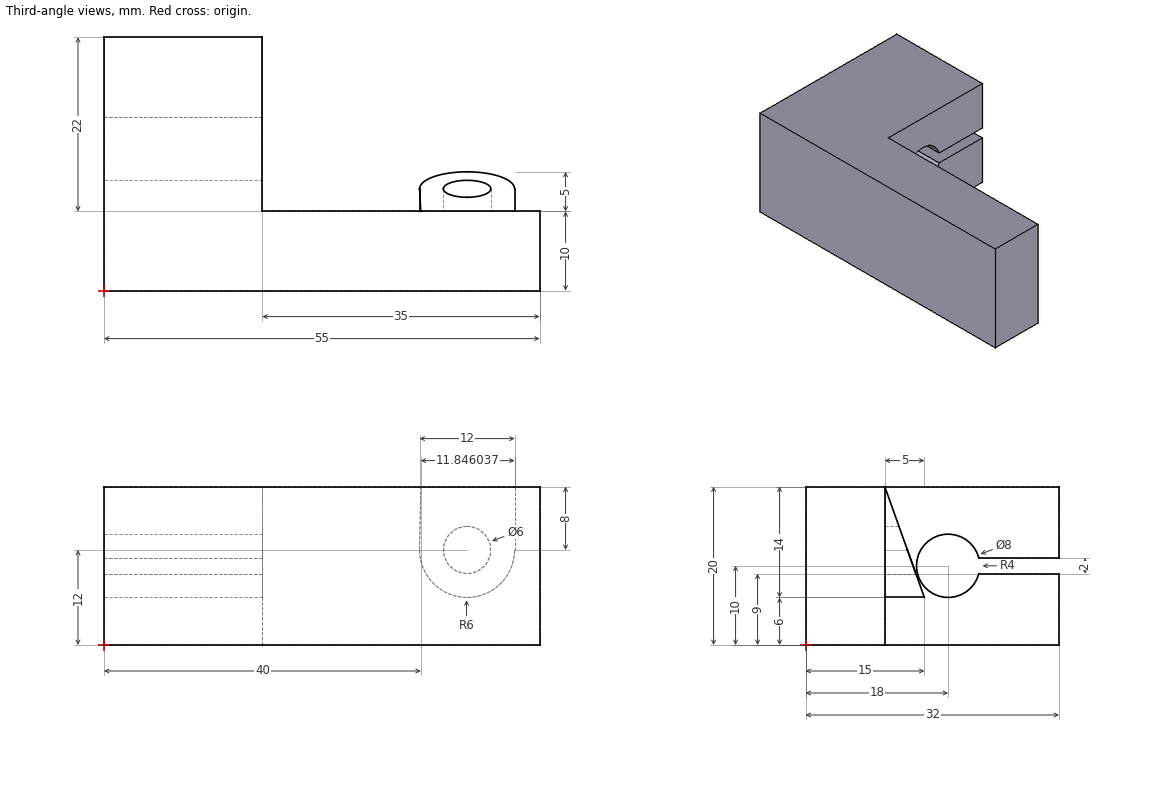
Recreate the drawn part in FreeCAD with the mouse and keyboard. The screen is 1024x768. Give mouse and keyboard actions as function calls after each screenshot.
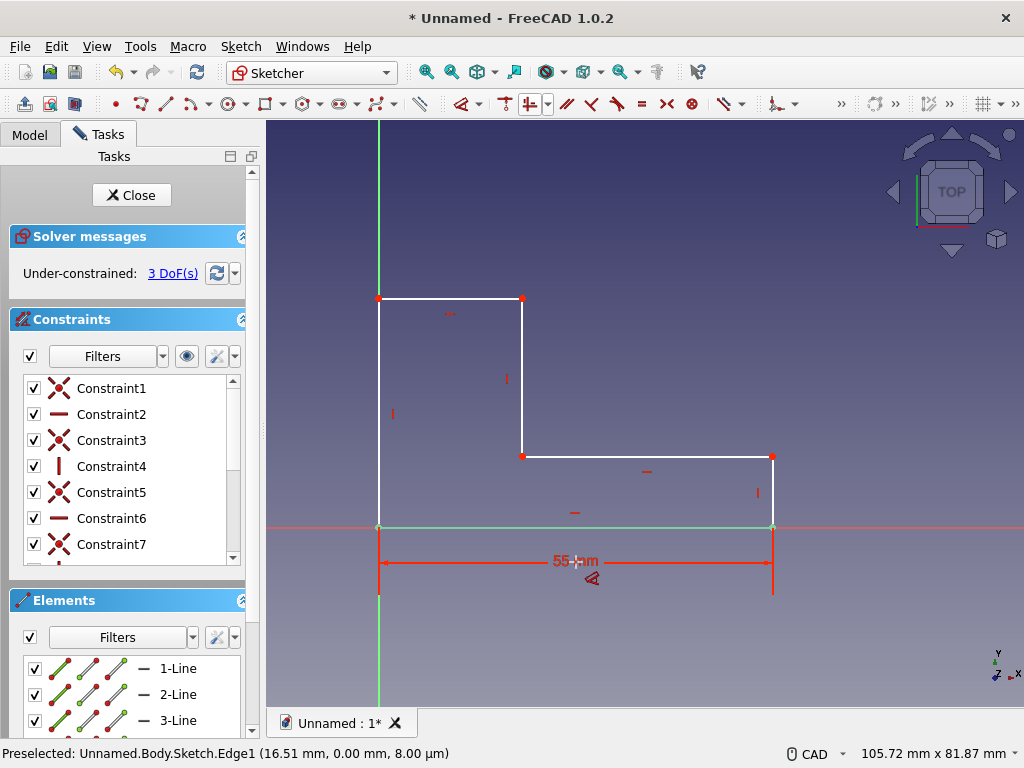
click(773, 506)
click(807, 492)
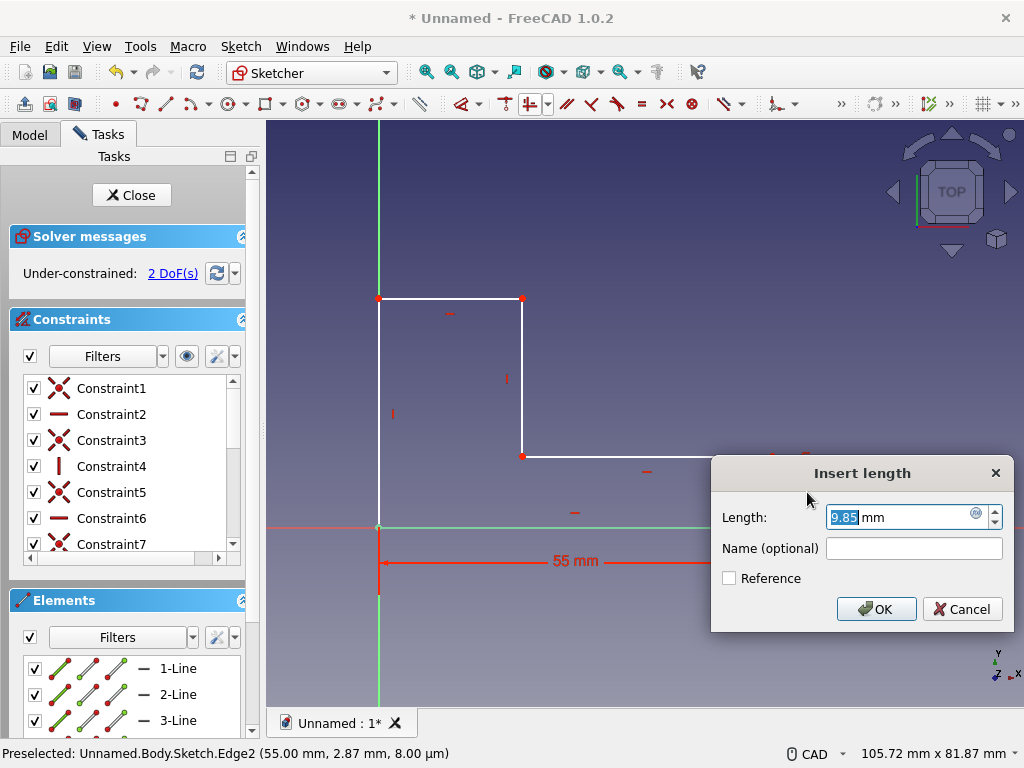
text(10)
key(Return)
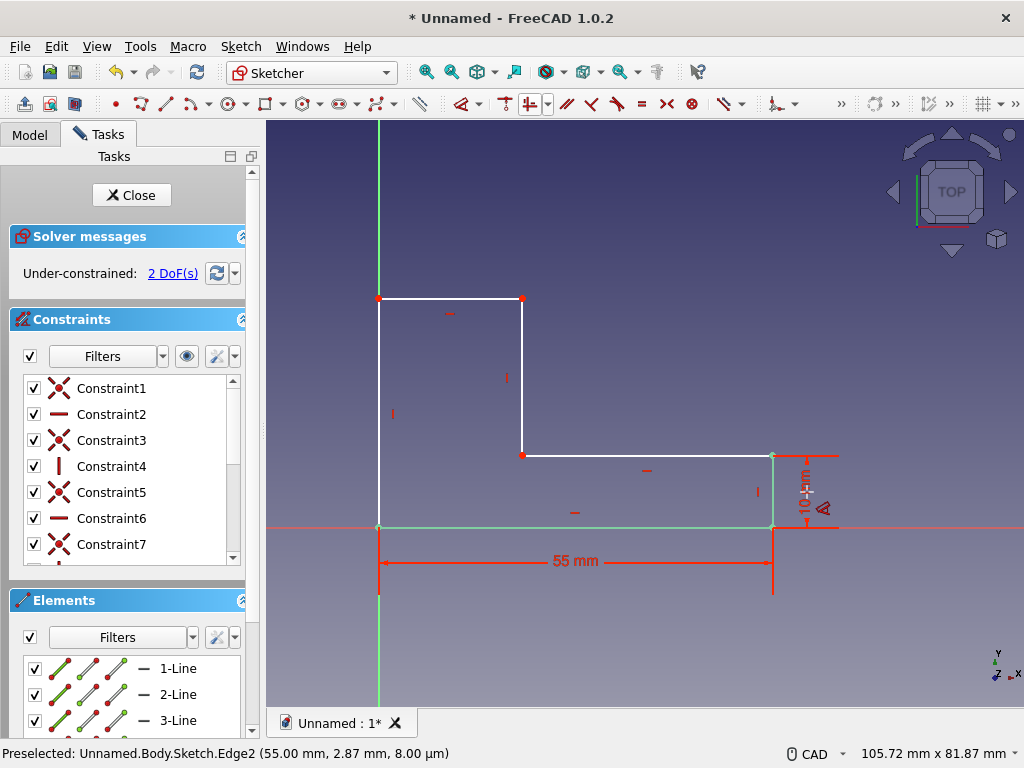
click(698, 456)
click(647, 490)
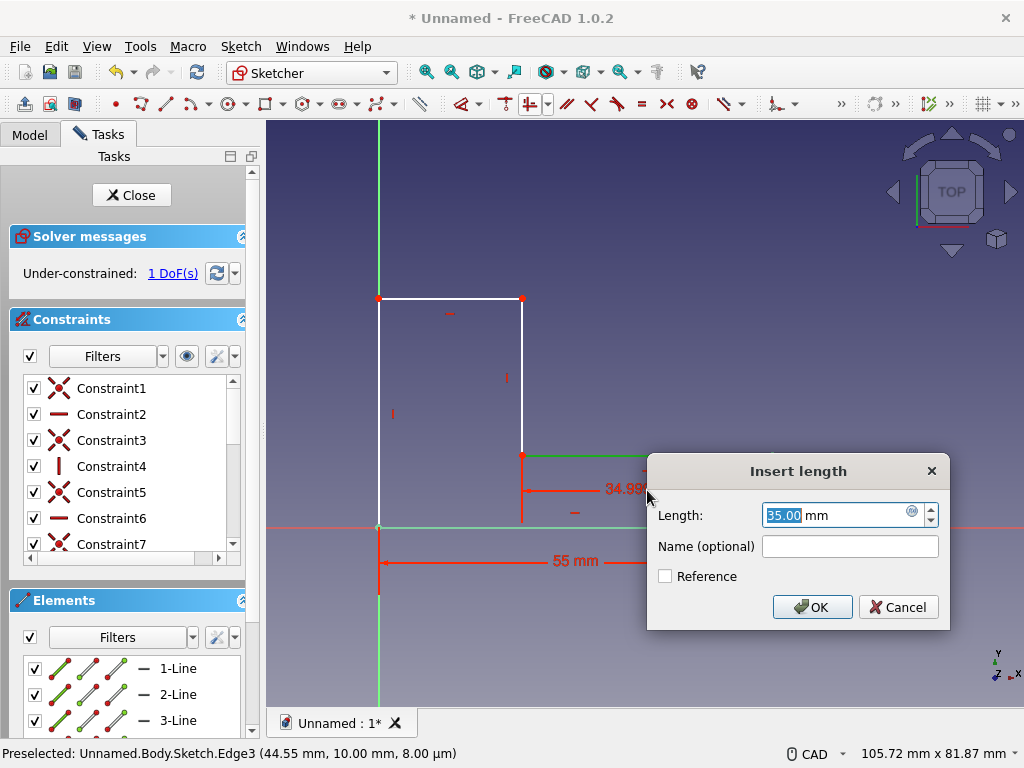
text(35)
key(Return)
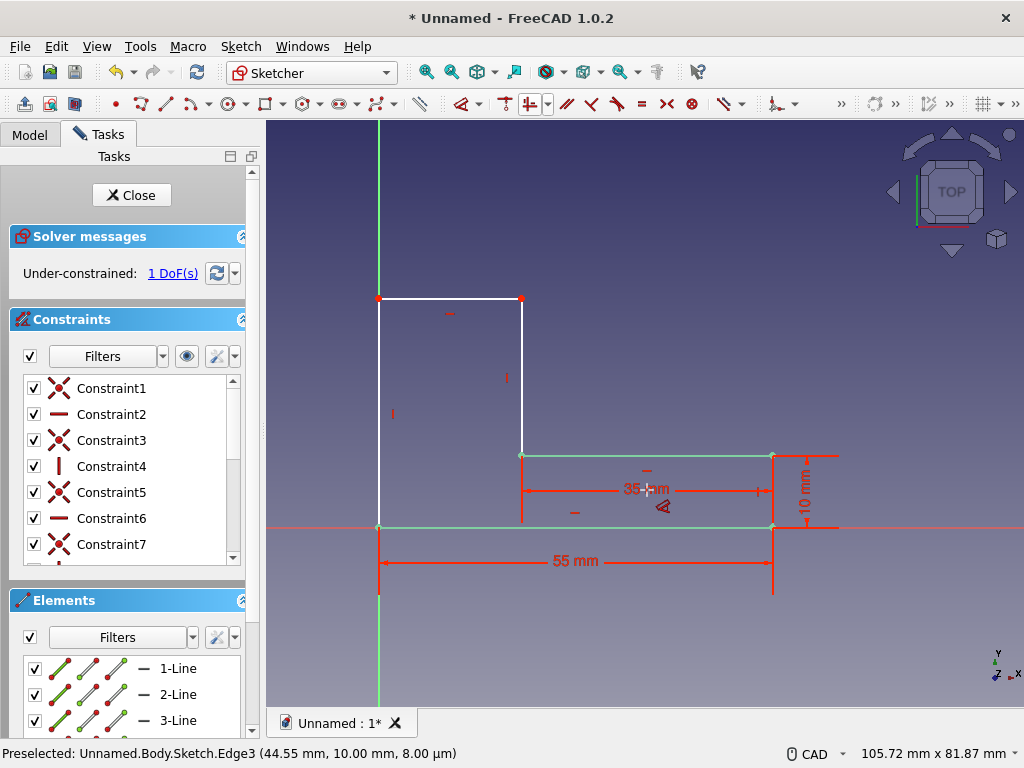
click(522, 409)
click(488, 377)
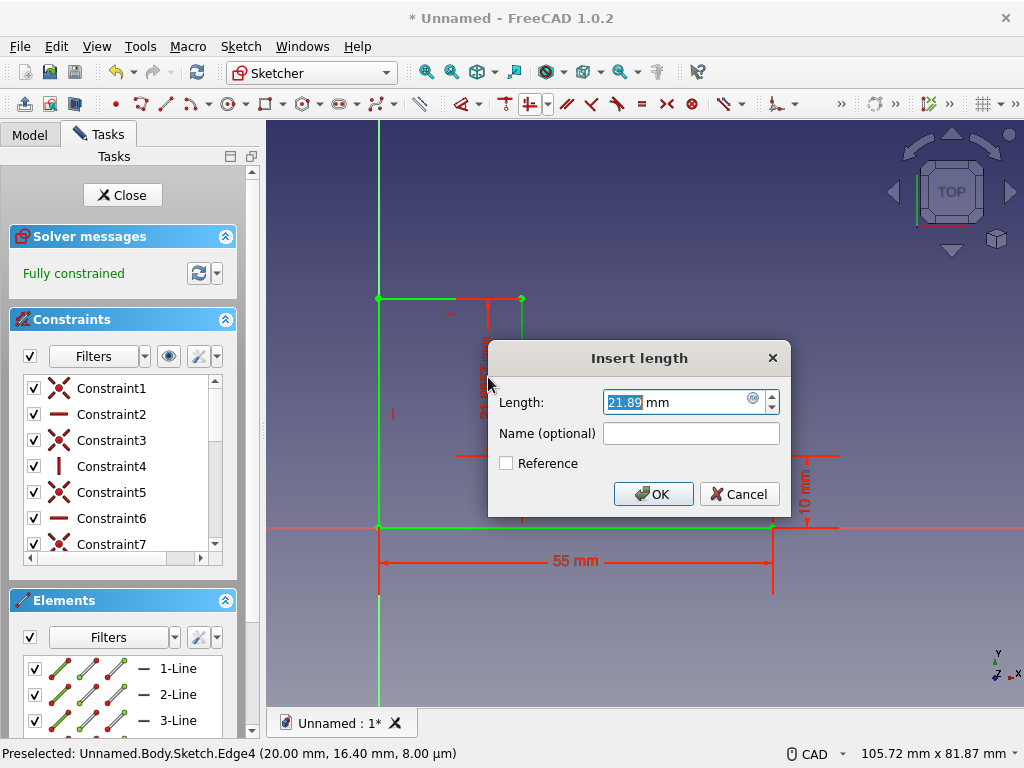
text(22)
key(Return)
key(Escape)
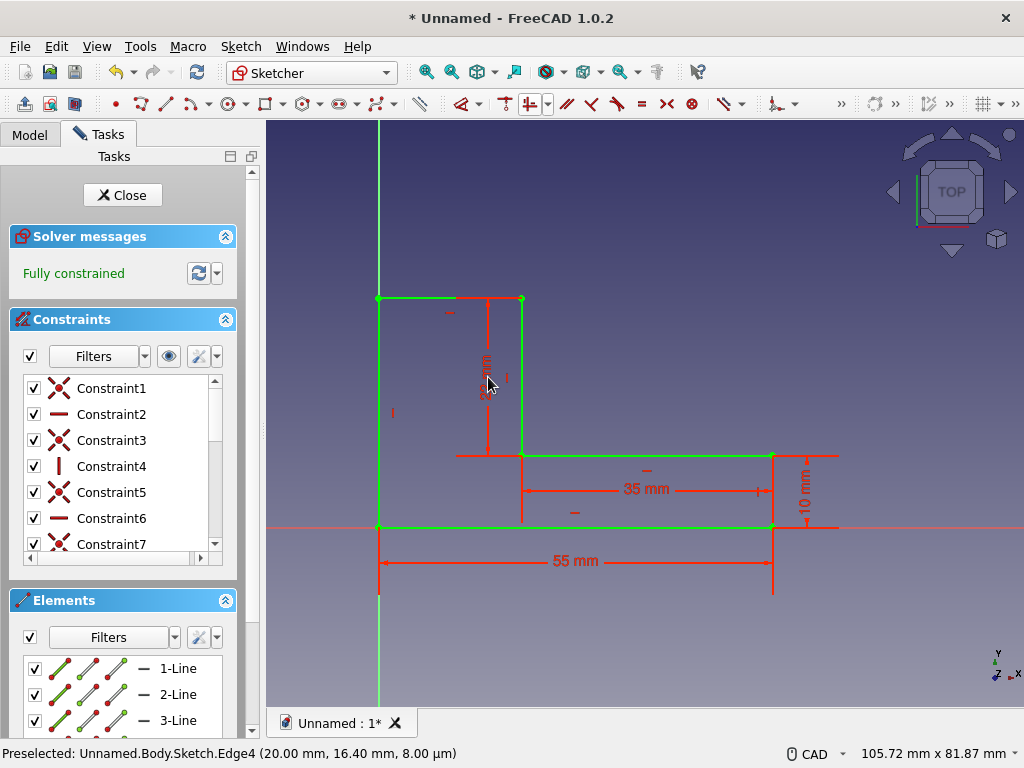
click(123, 195)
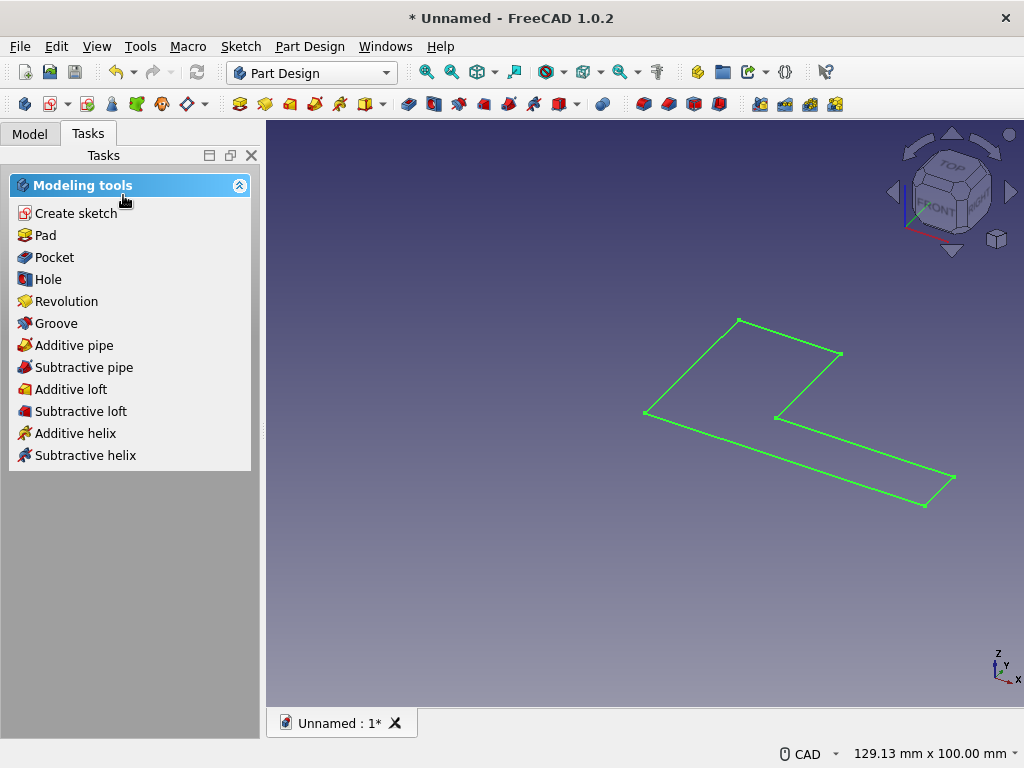
click(240, 104)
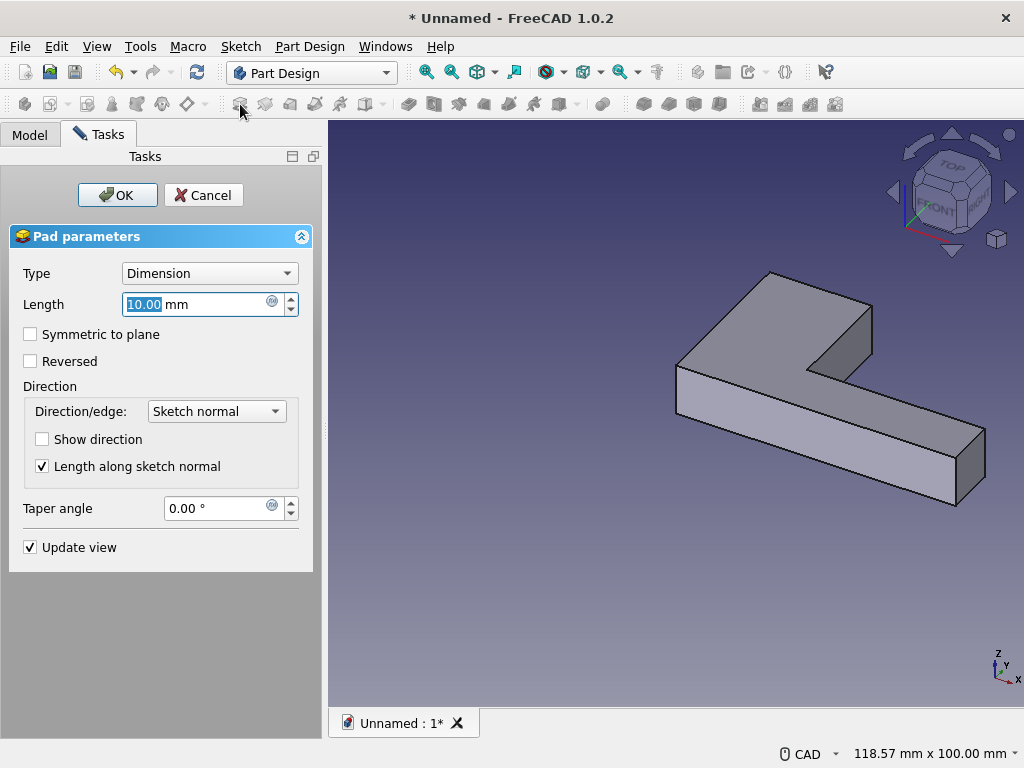
text(20)
key(Tab)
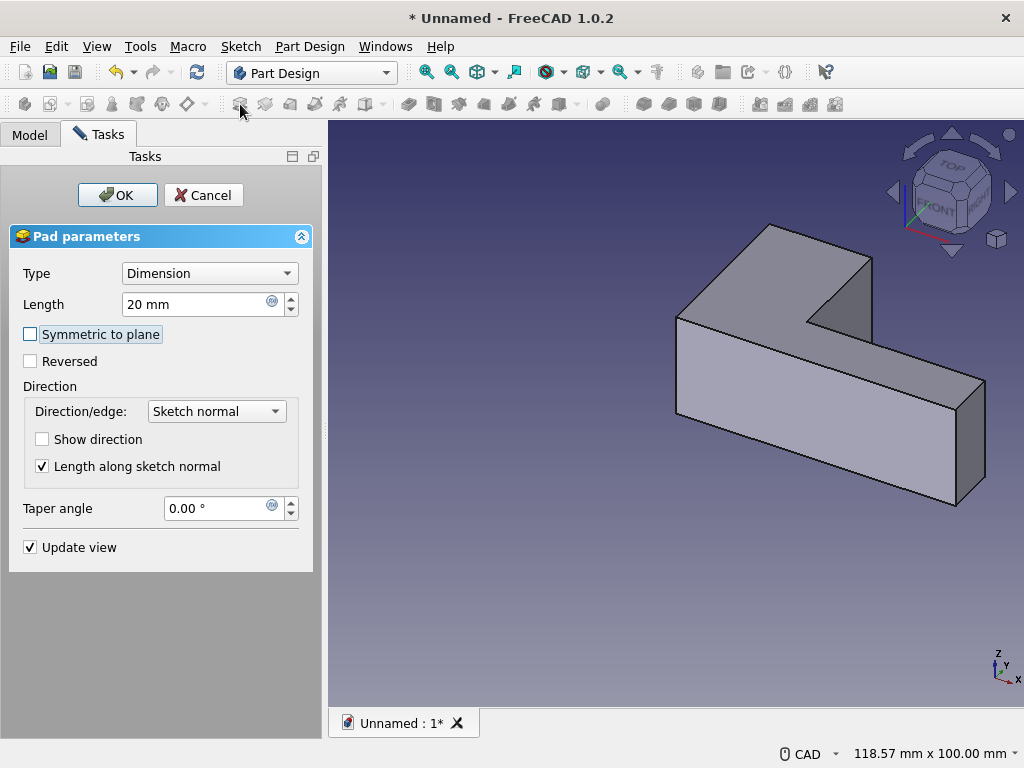
click(118, 195)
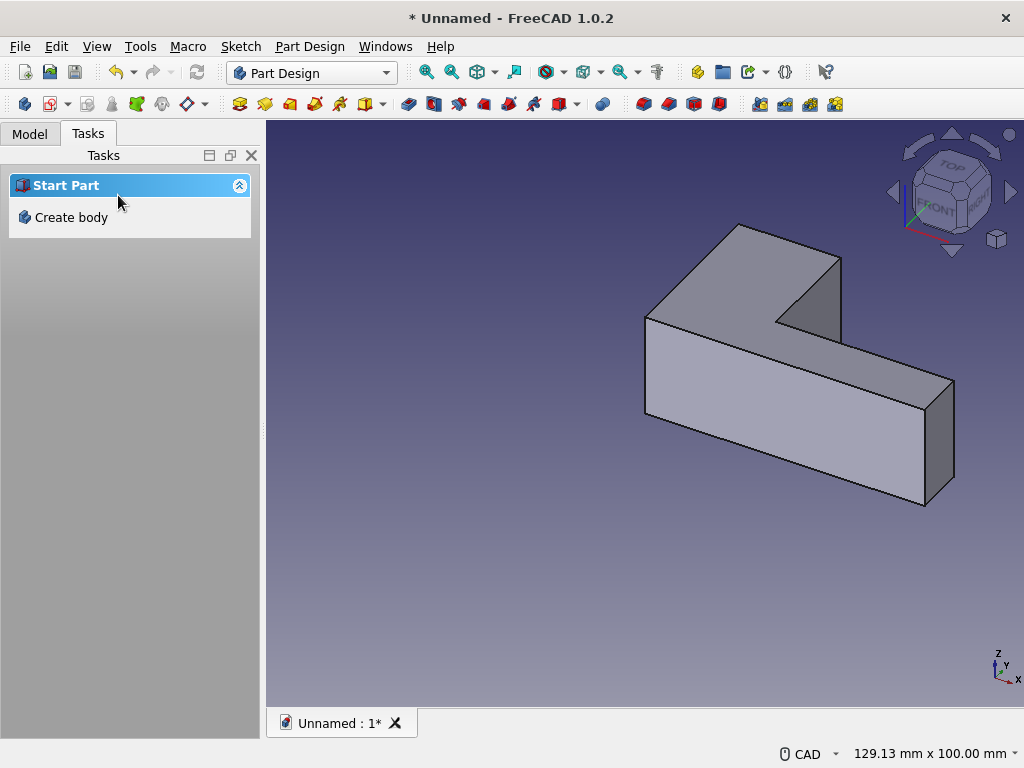
click(818, 314)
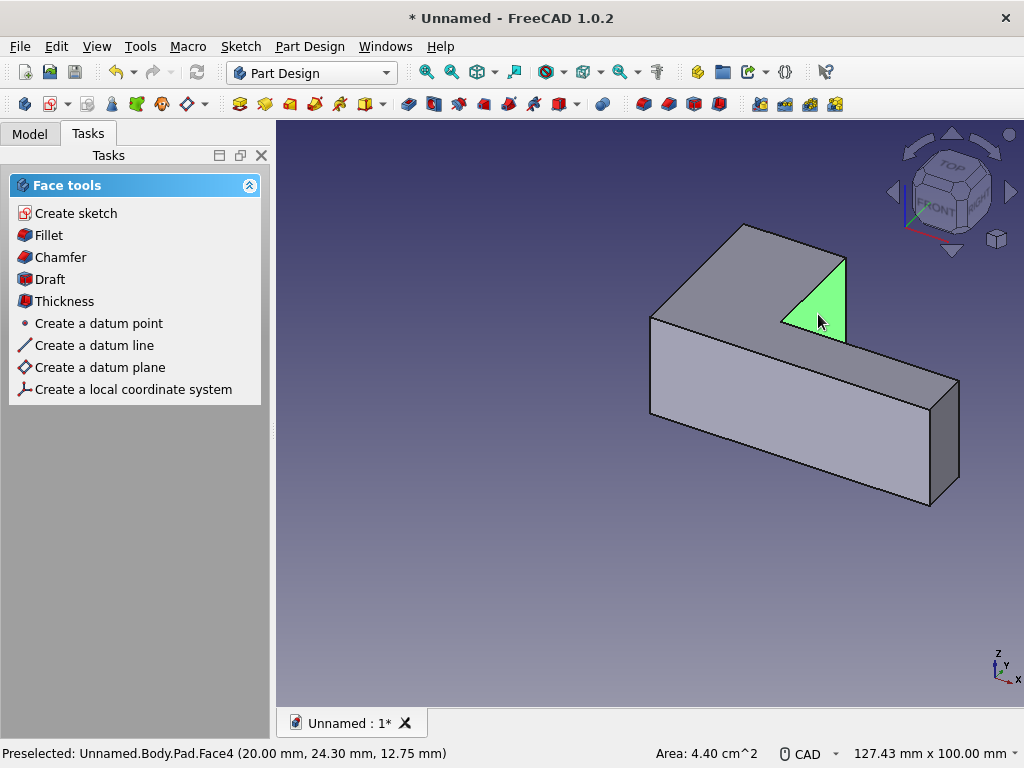
click(50, 104)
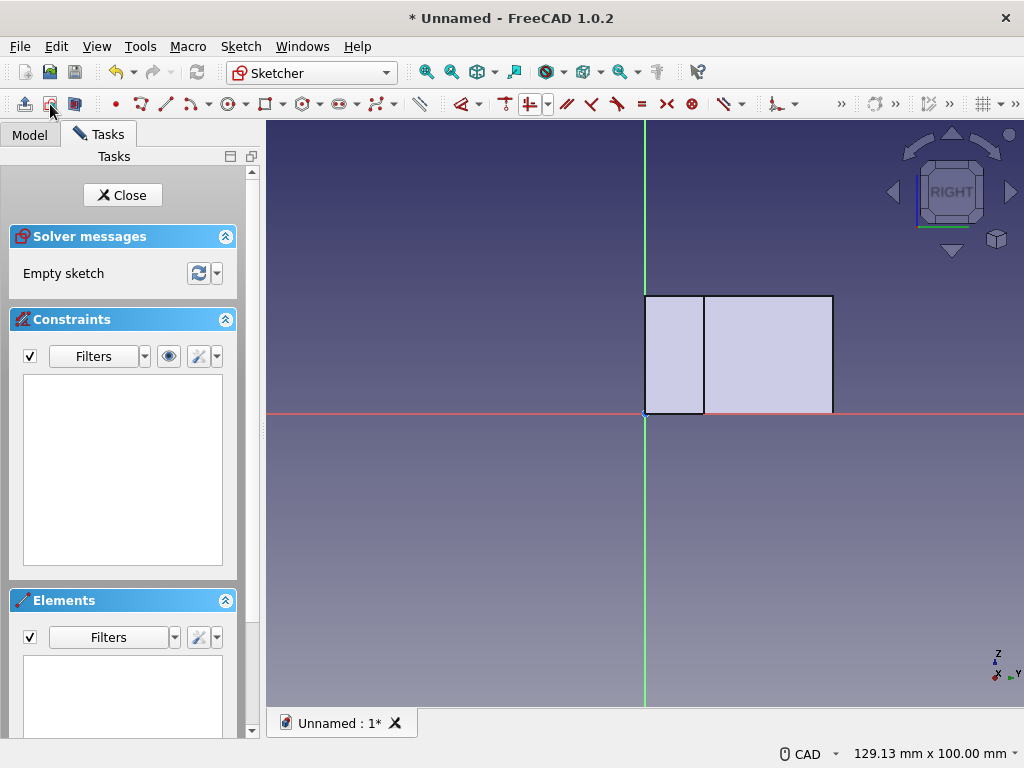
scroll(778, 346, up, 10)